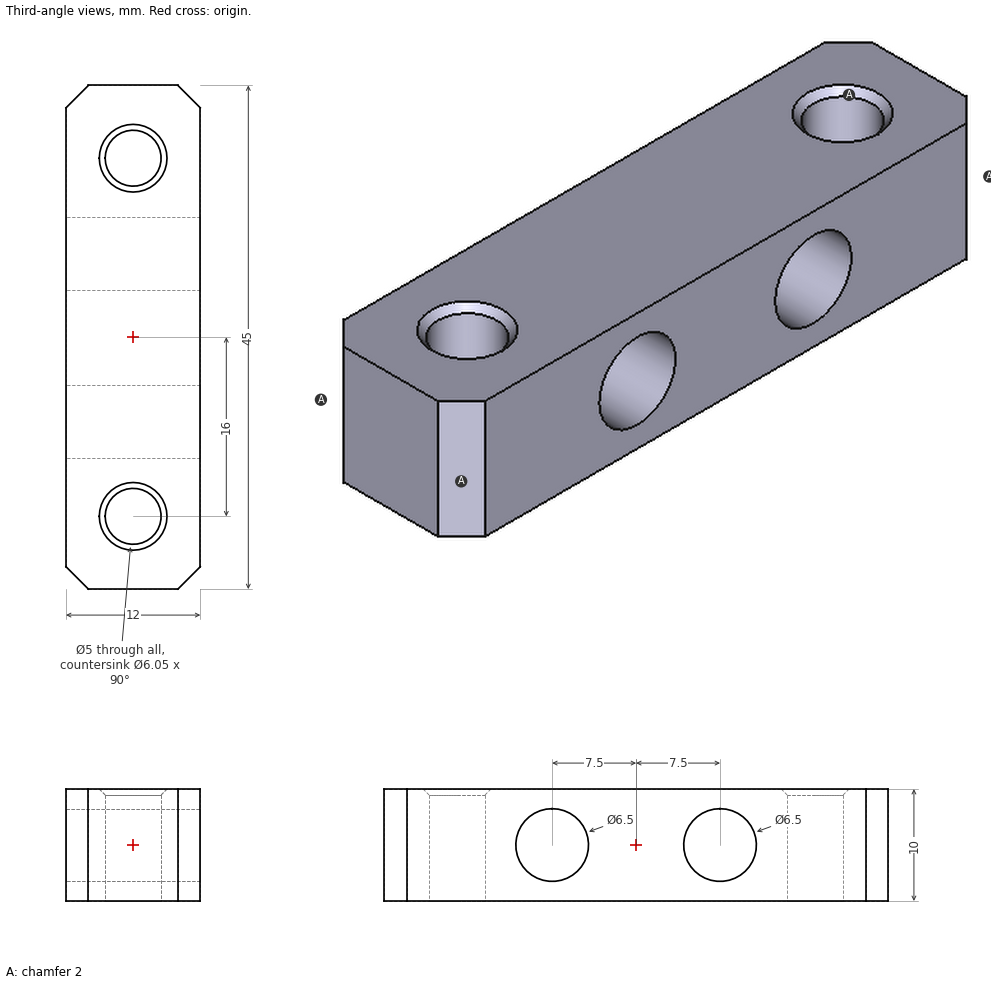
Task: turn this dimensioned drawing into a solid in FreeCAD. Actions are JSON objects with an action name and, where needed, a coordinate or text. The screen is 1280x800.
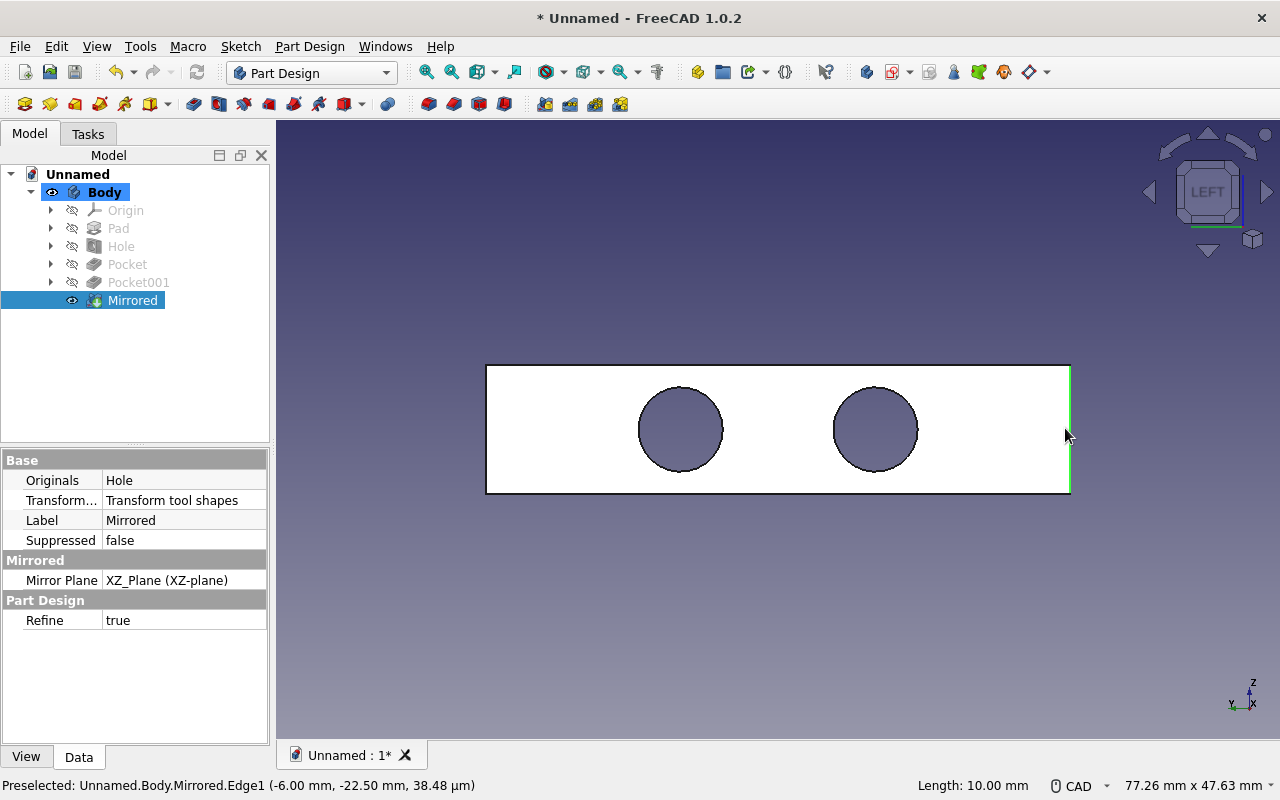
{"action": "left_click", "coordinate": [486, 428], "text": "ctrl"}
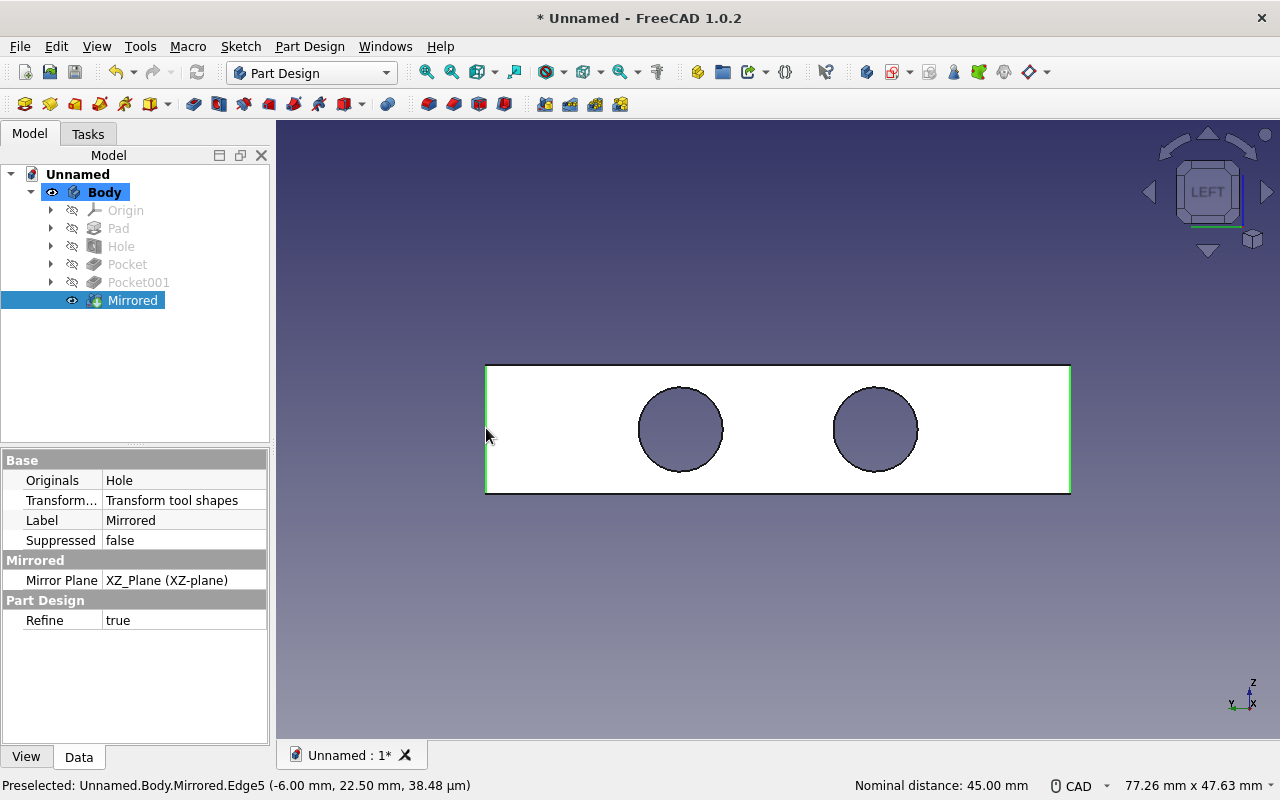
{"action": "key", "text": "0"}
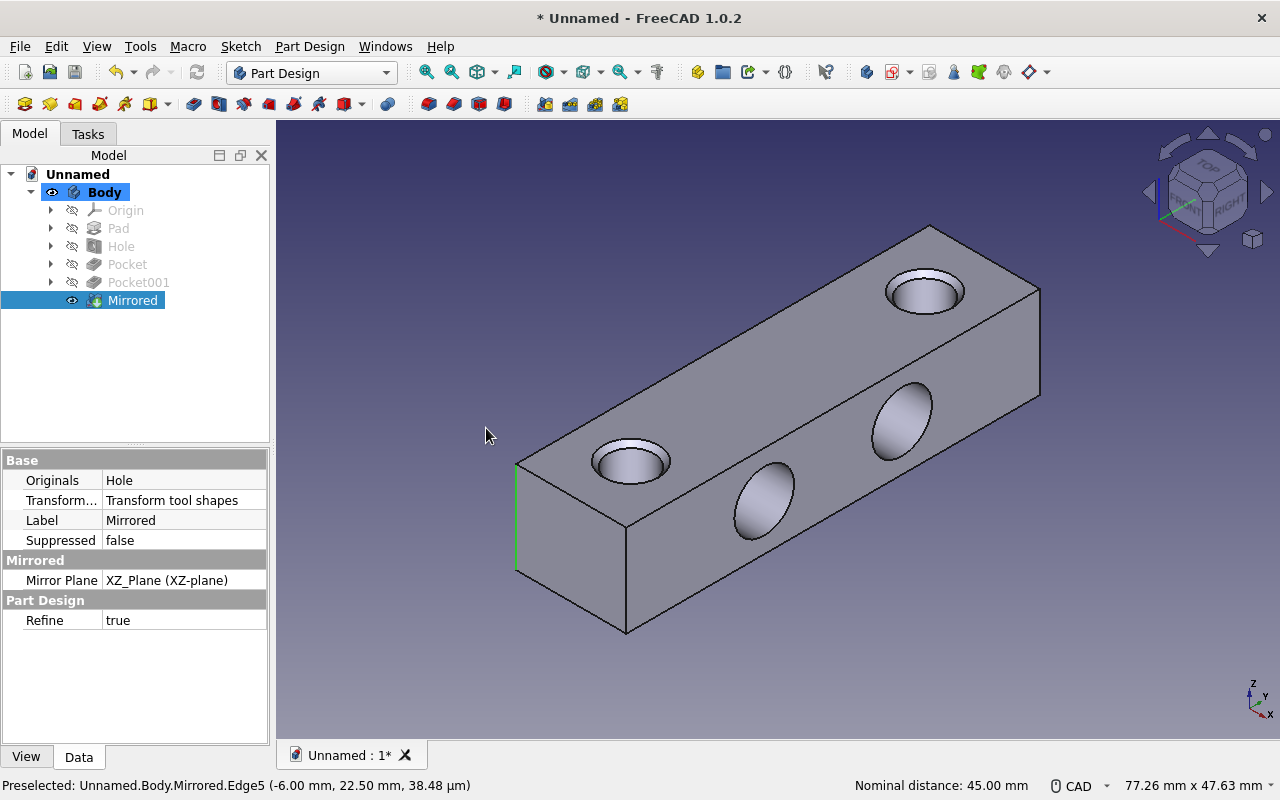
{"action": "left_click", "coordinate": [626, 580], "text": "ctrl"}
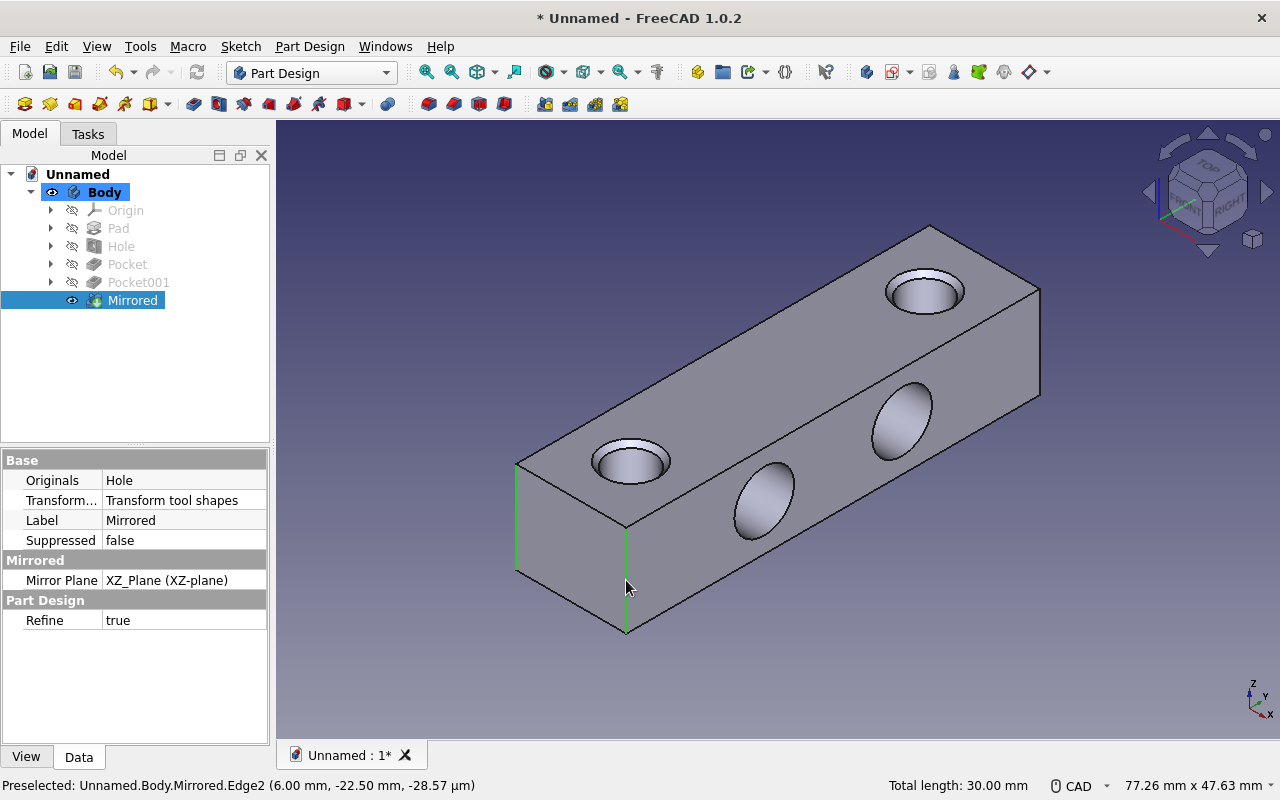
{"action": "key", "text": "2"}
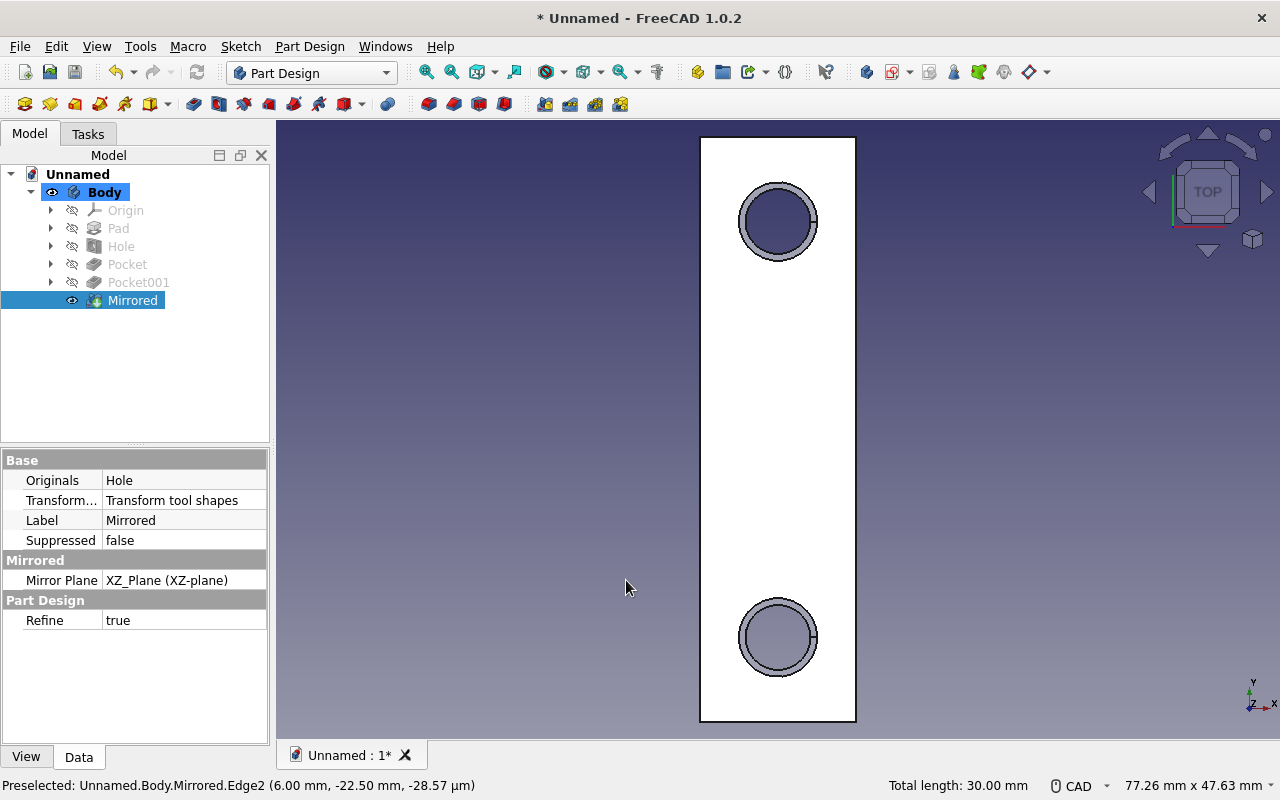
{"action": "key", "text": "1"}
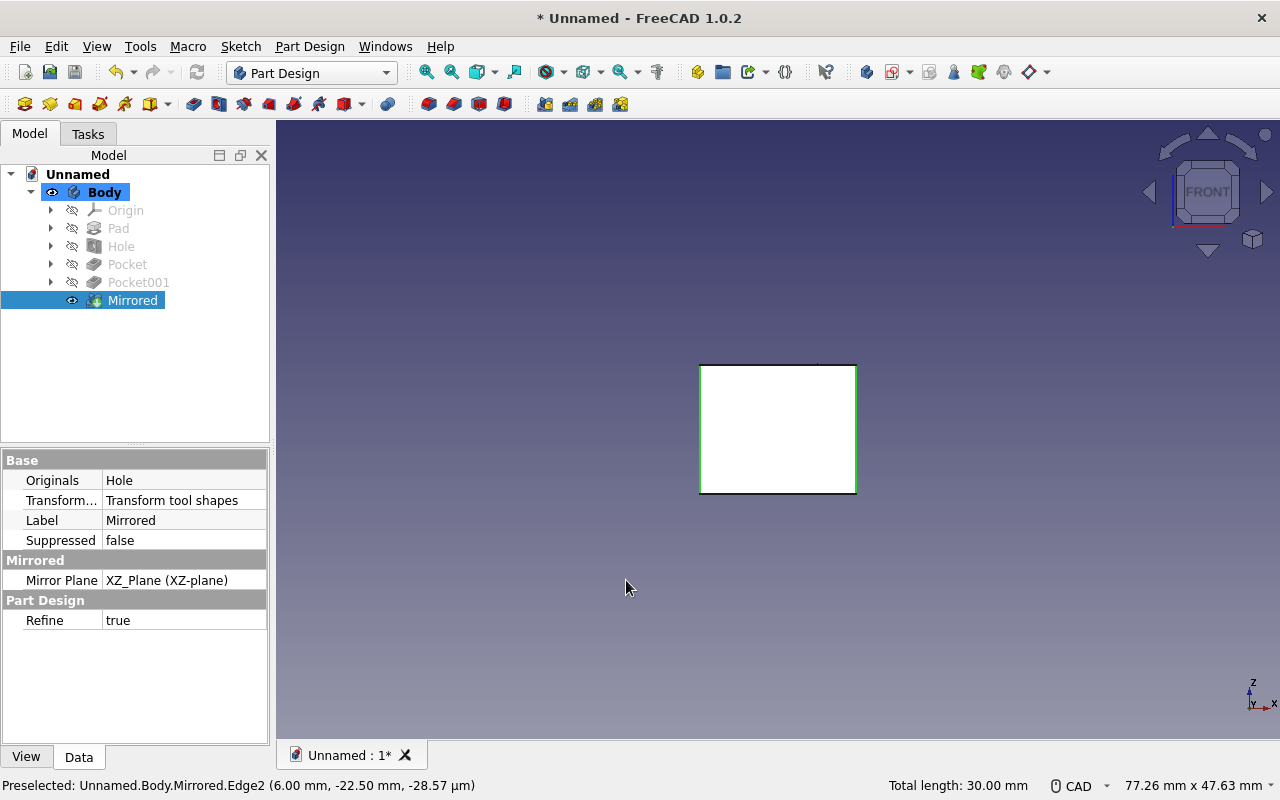
{"action": "key", "text": "v f"}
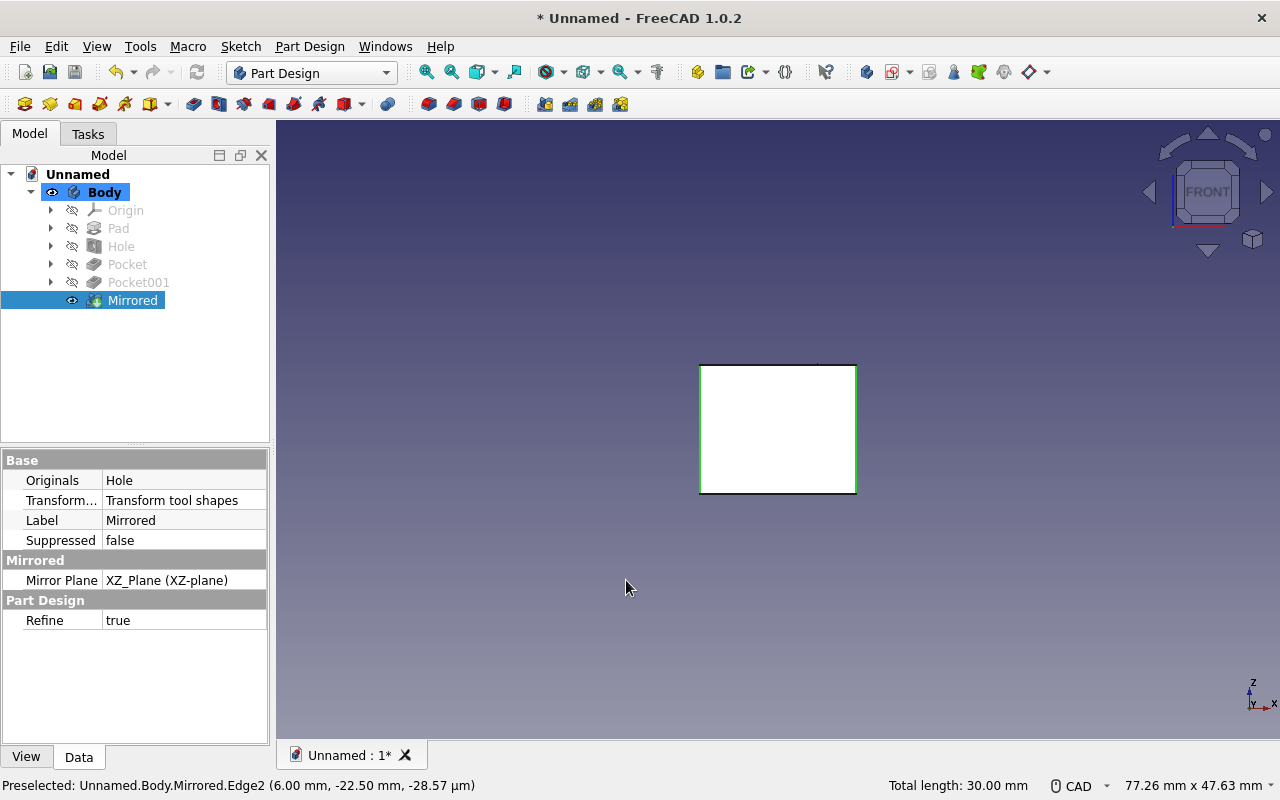
{"action": "key", "text": "3"}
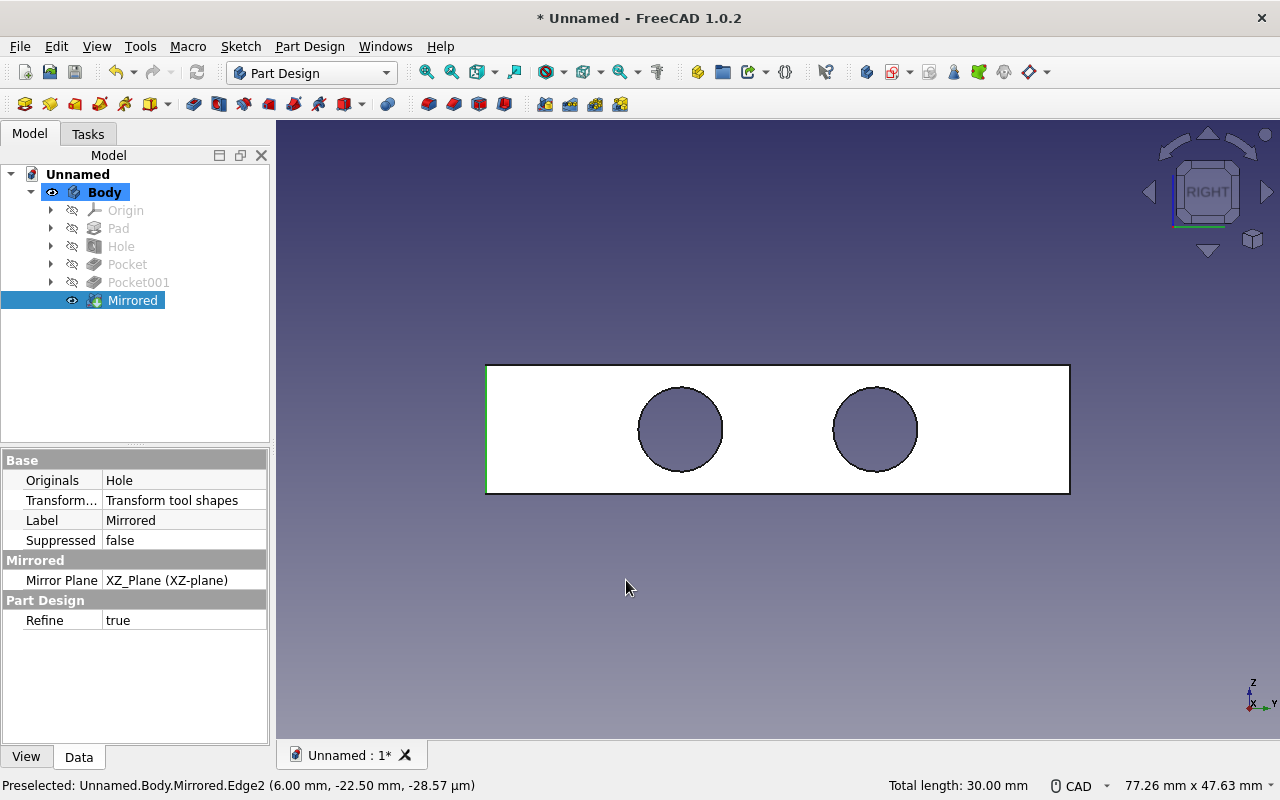
{"action": "left_click", "coordinate": [1070, 428], "text": "ctrl"}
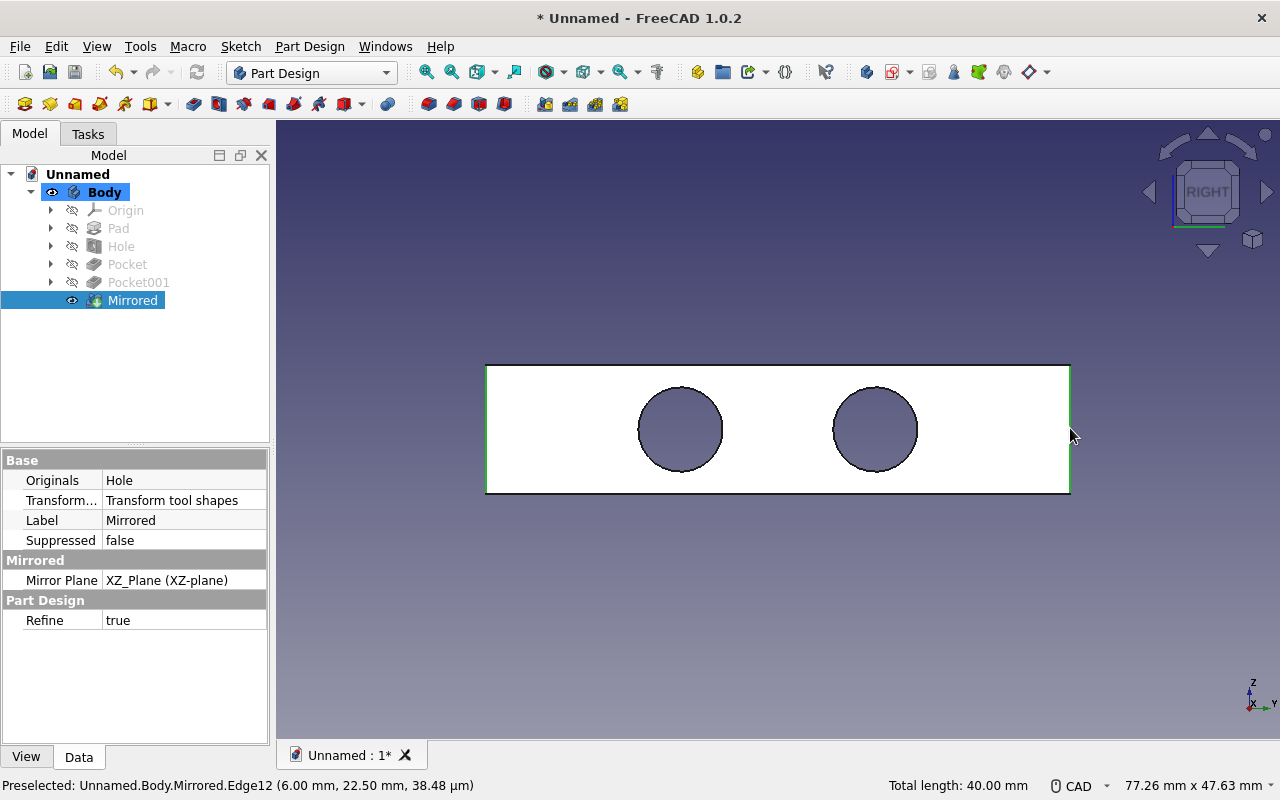
{"action": "left_click", "coordinate": [454, 104]}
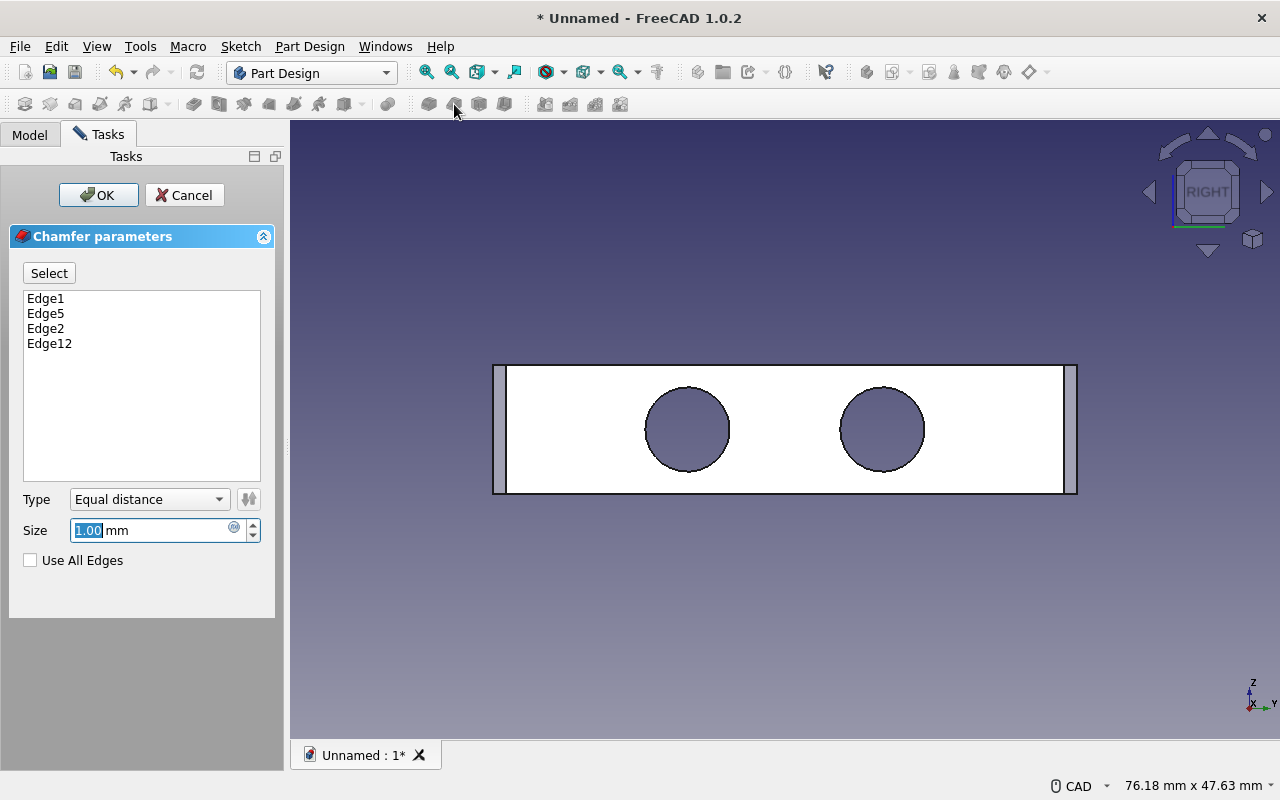
{"action": "type", "text": "2"}
{"action": "key", "text": "Tab"}